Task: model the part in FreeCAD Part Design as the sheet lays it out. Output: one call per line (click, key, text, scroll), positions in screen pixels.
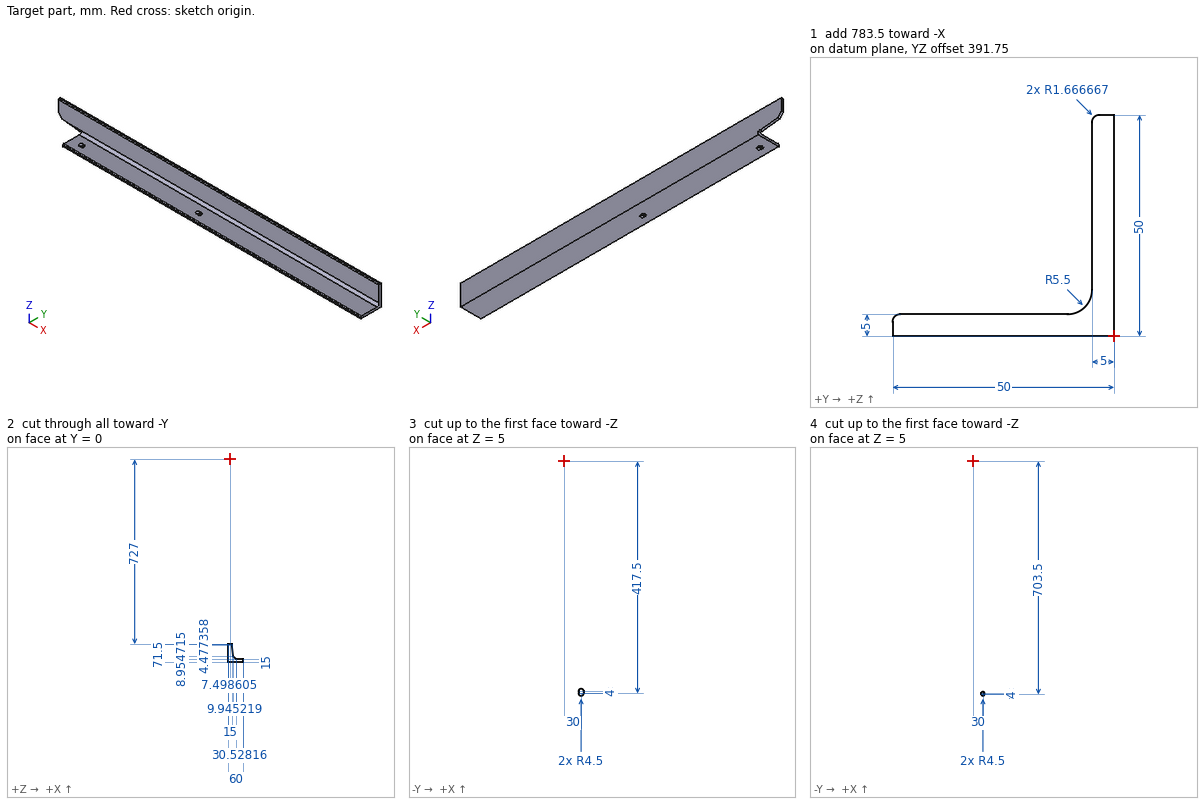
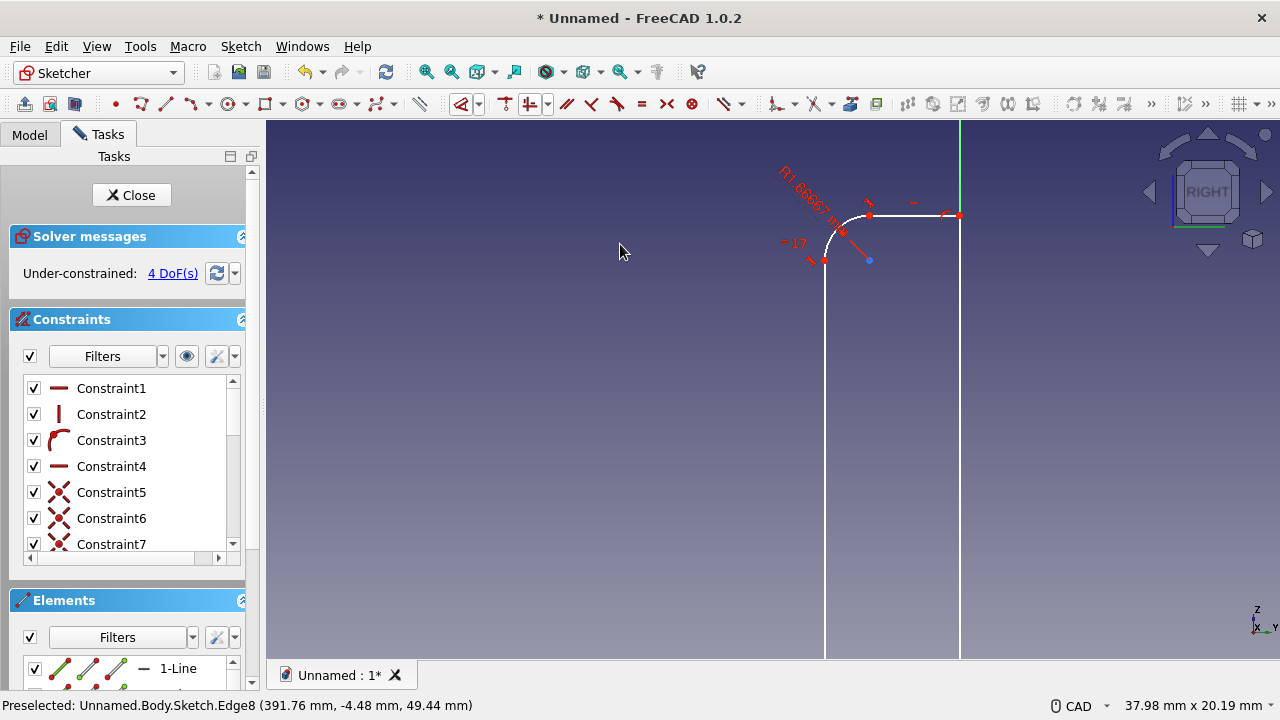
scroll(839, 229, down, 7)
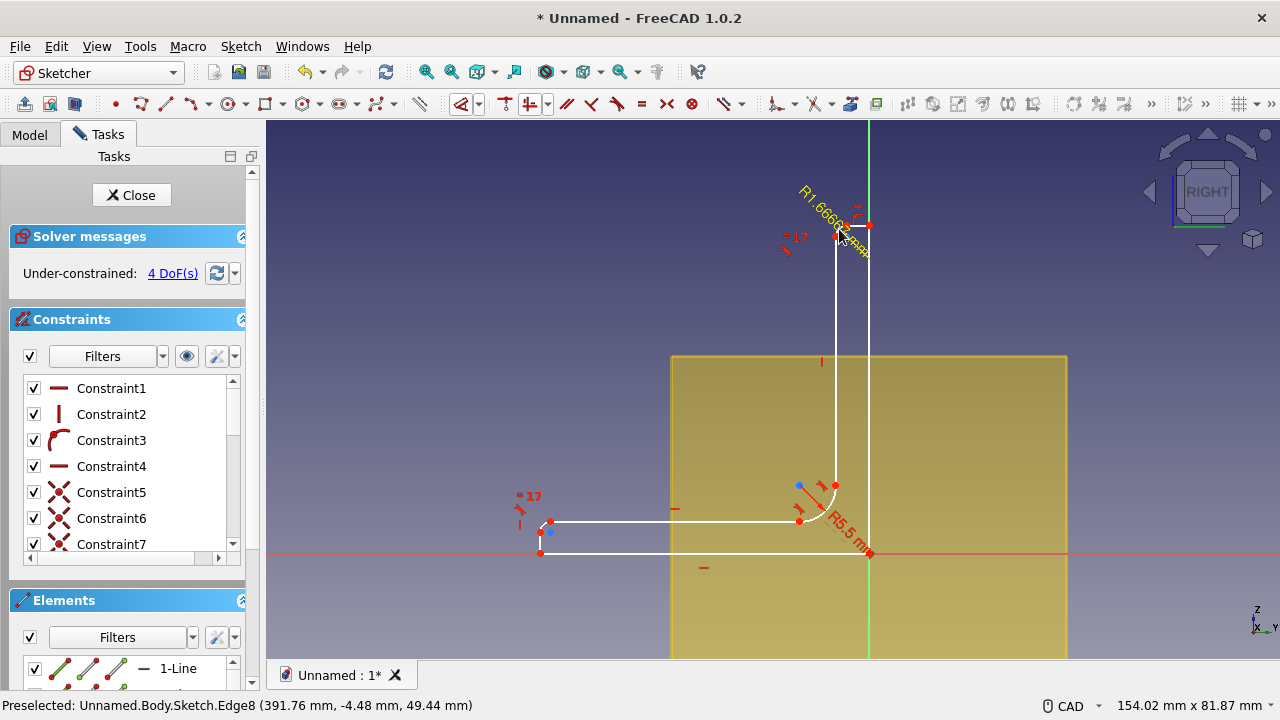
click(869, 324)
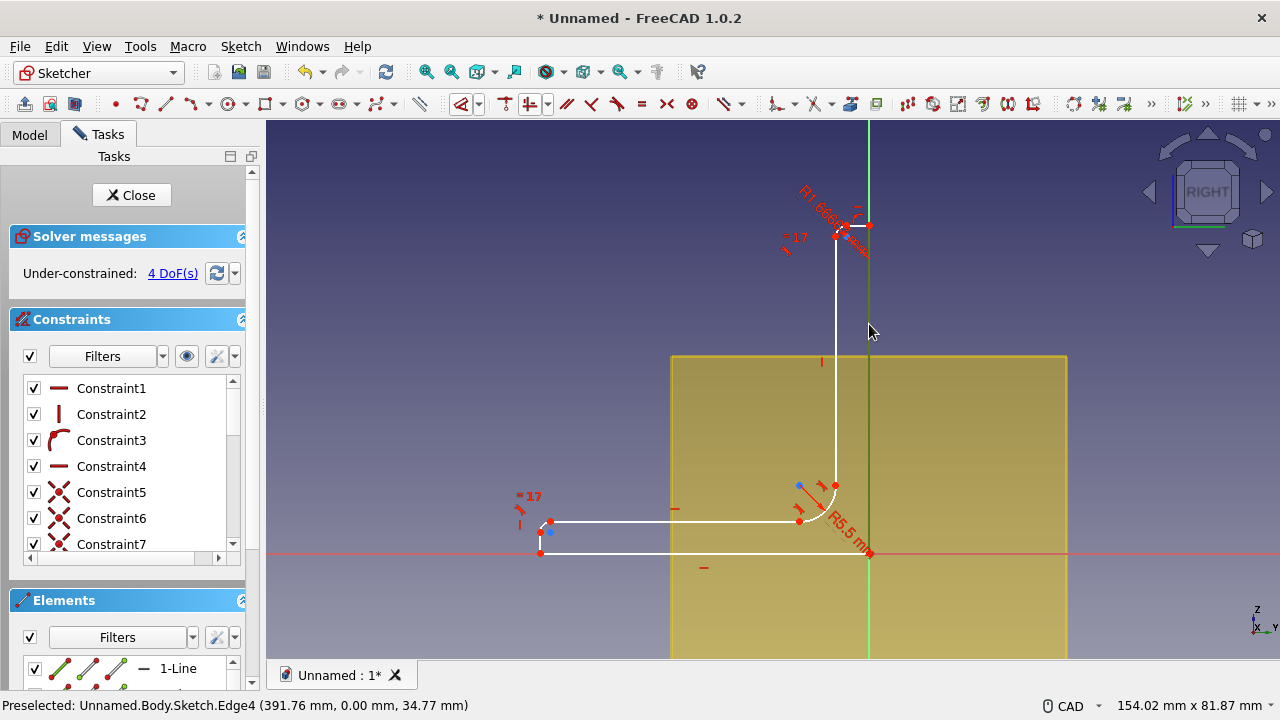
key(i)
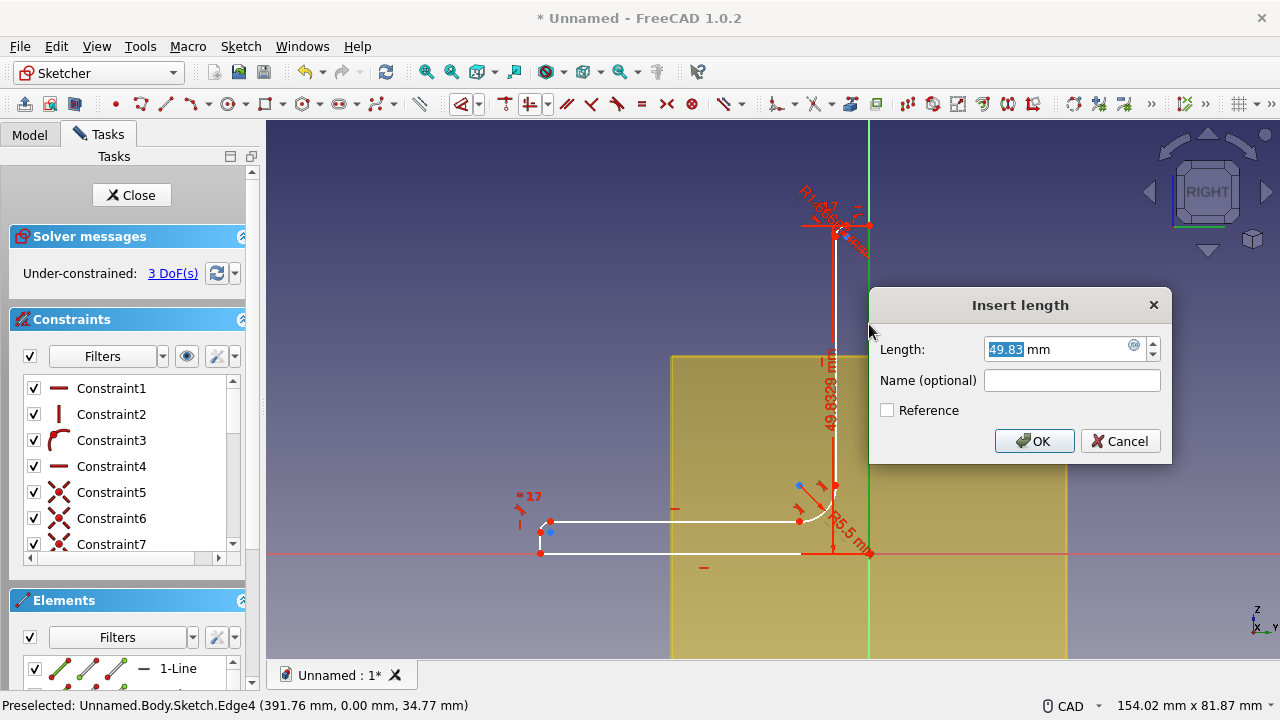
text(50)
key(Return)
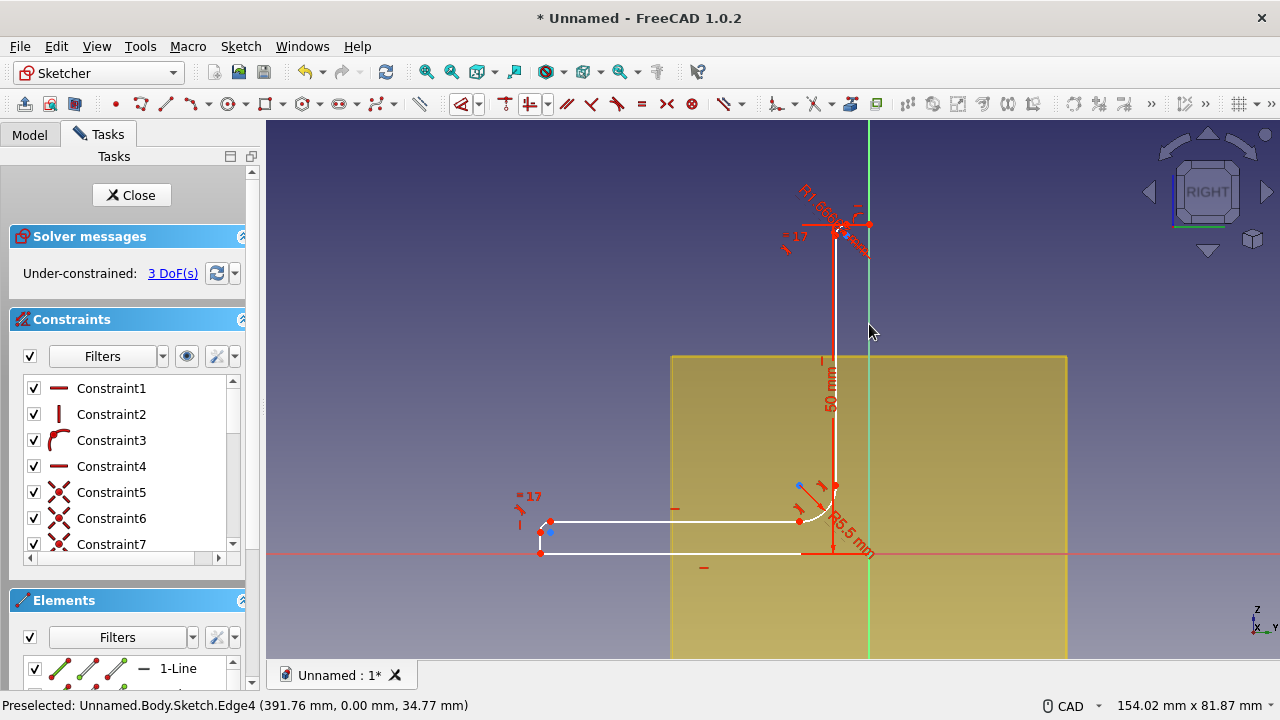
click(770, 554)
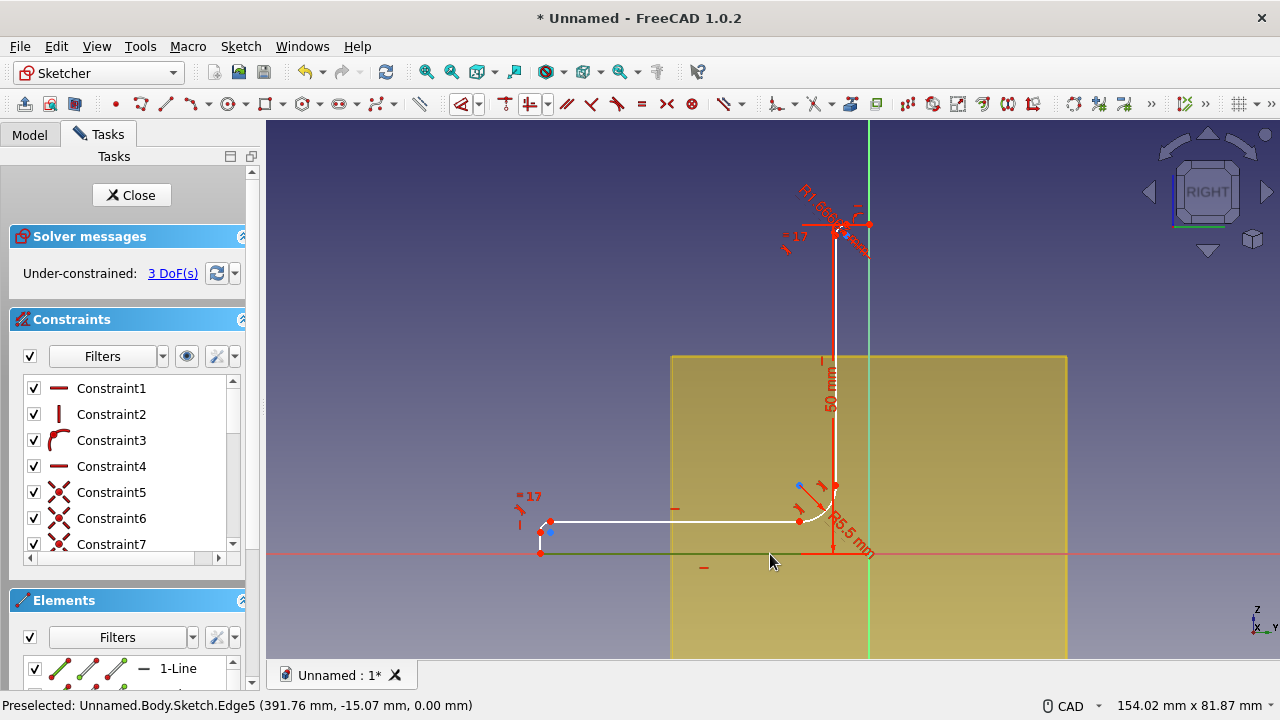
key(l)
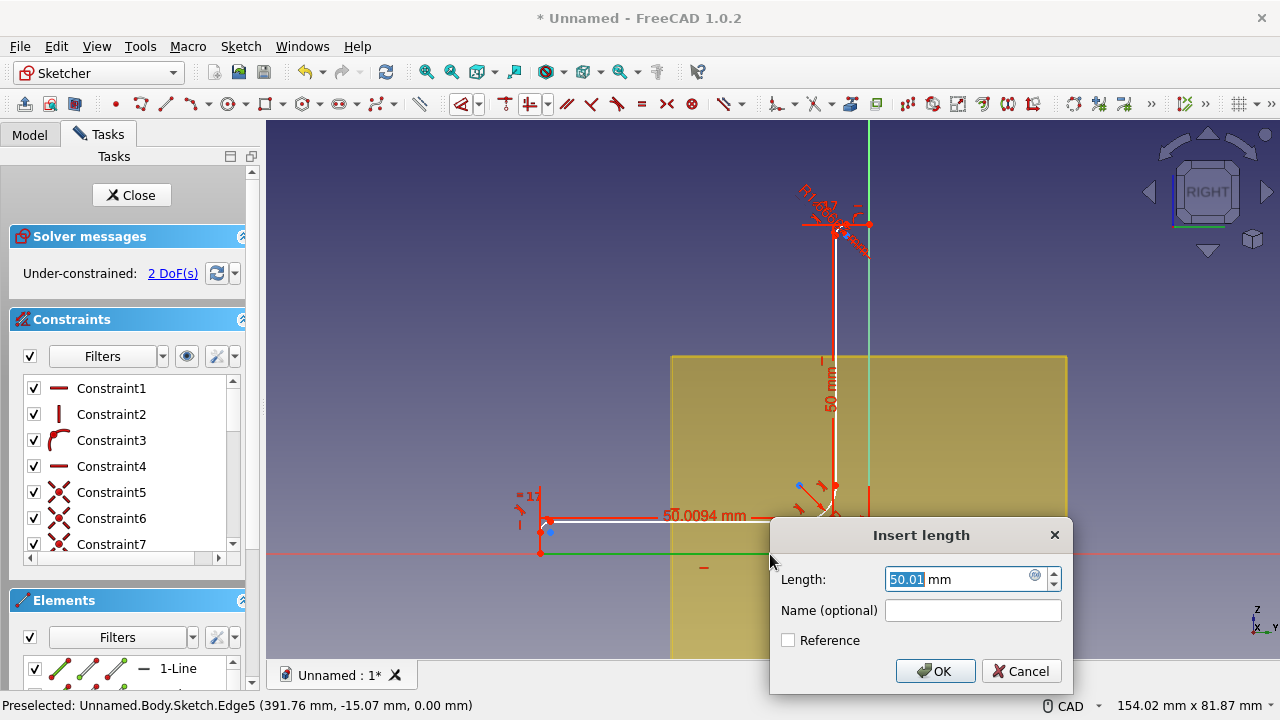
text(50)
key(Return)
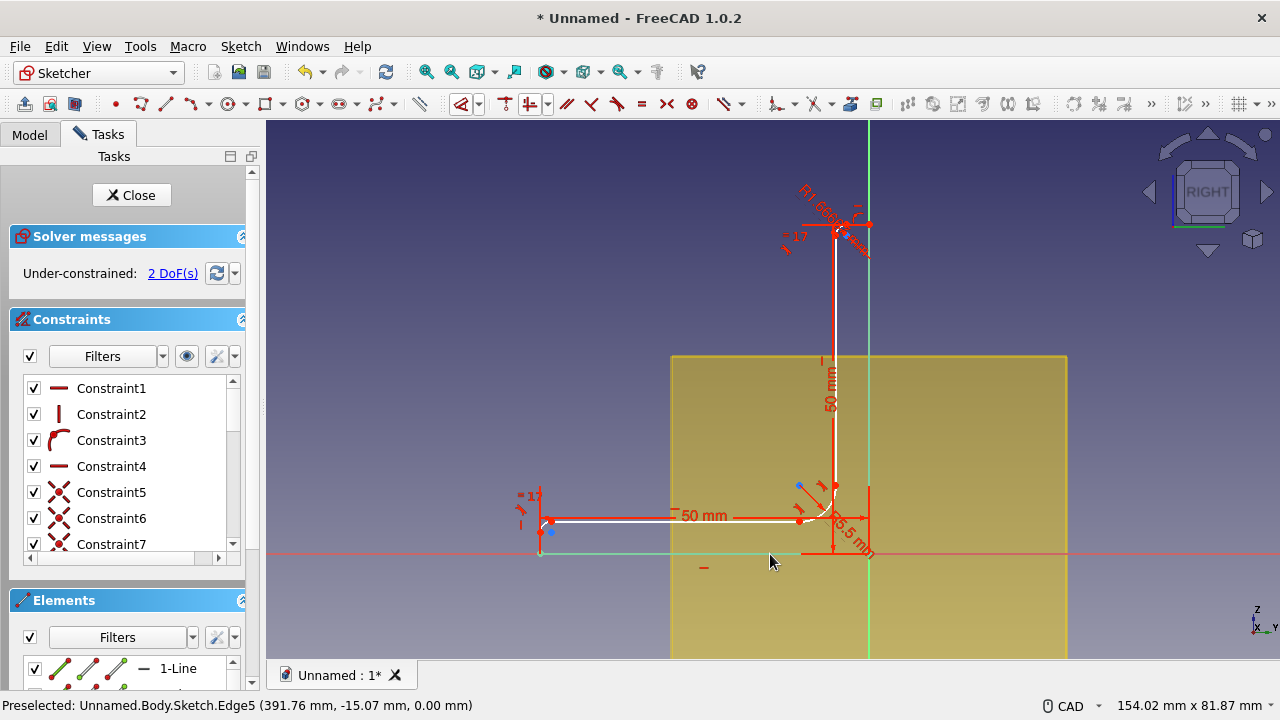
click(551, 522)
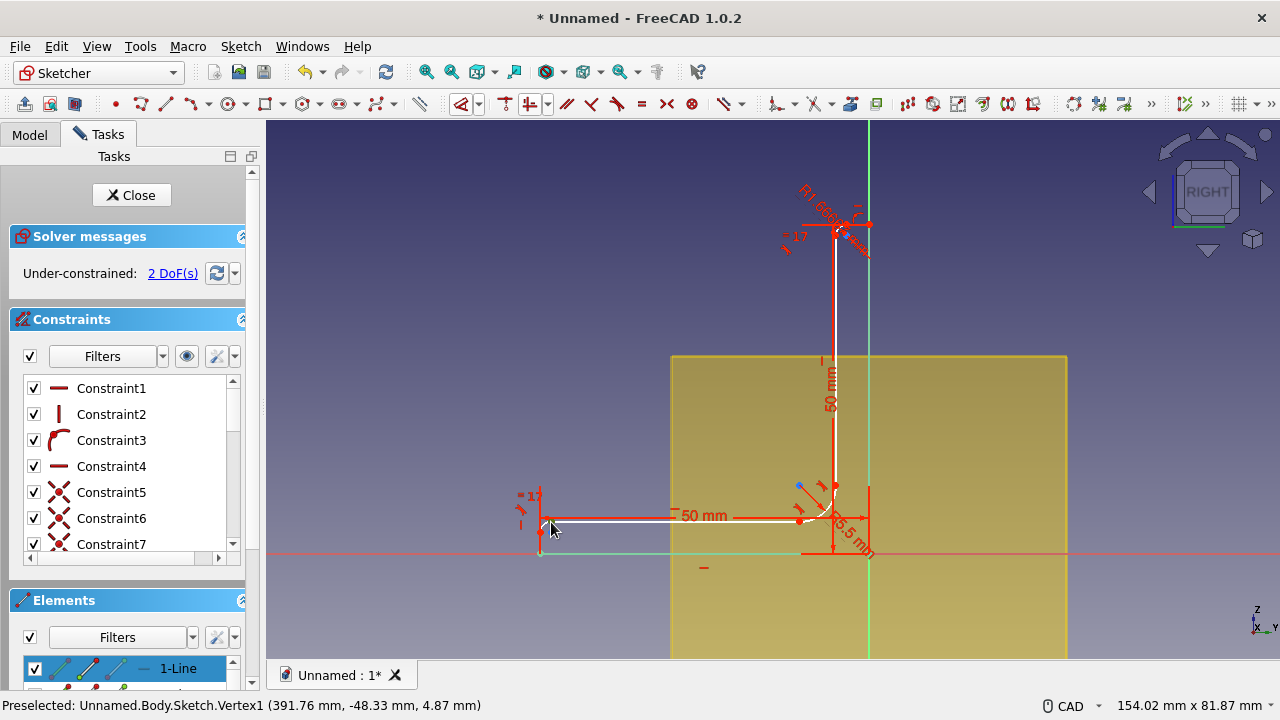
key(i)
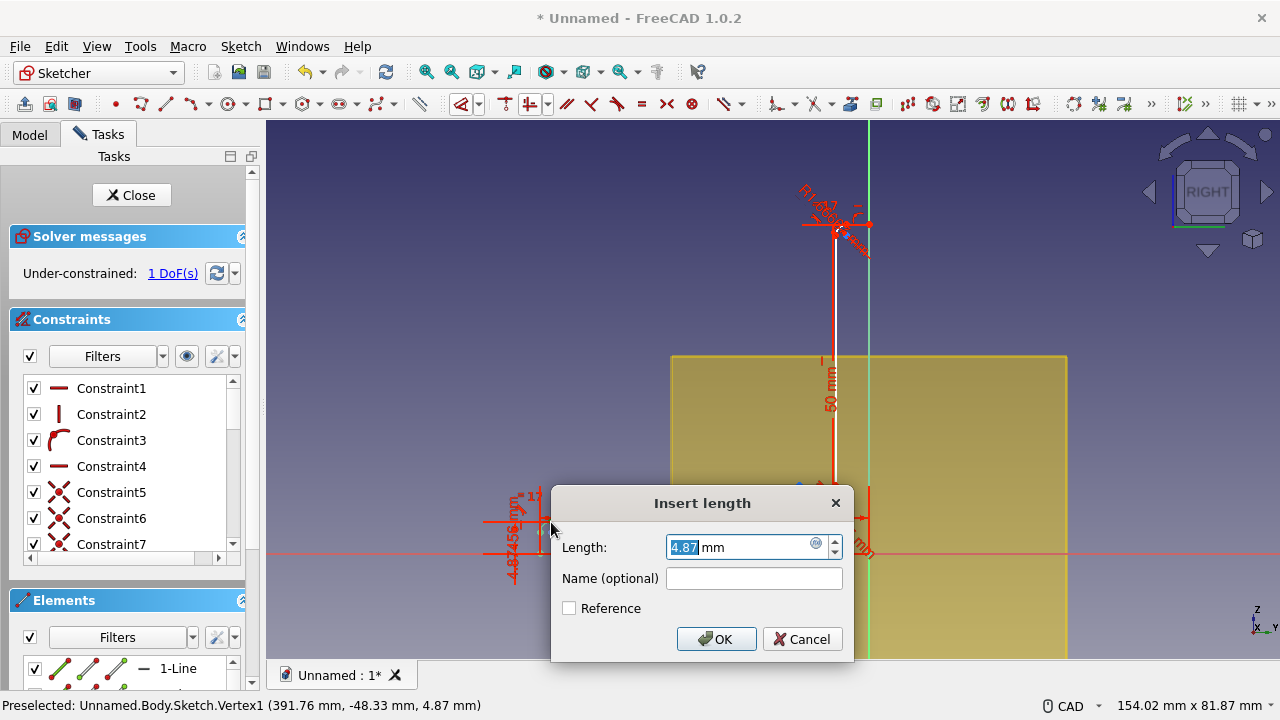
text(5)
key(Return)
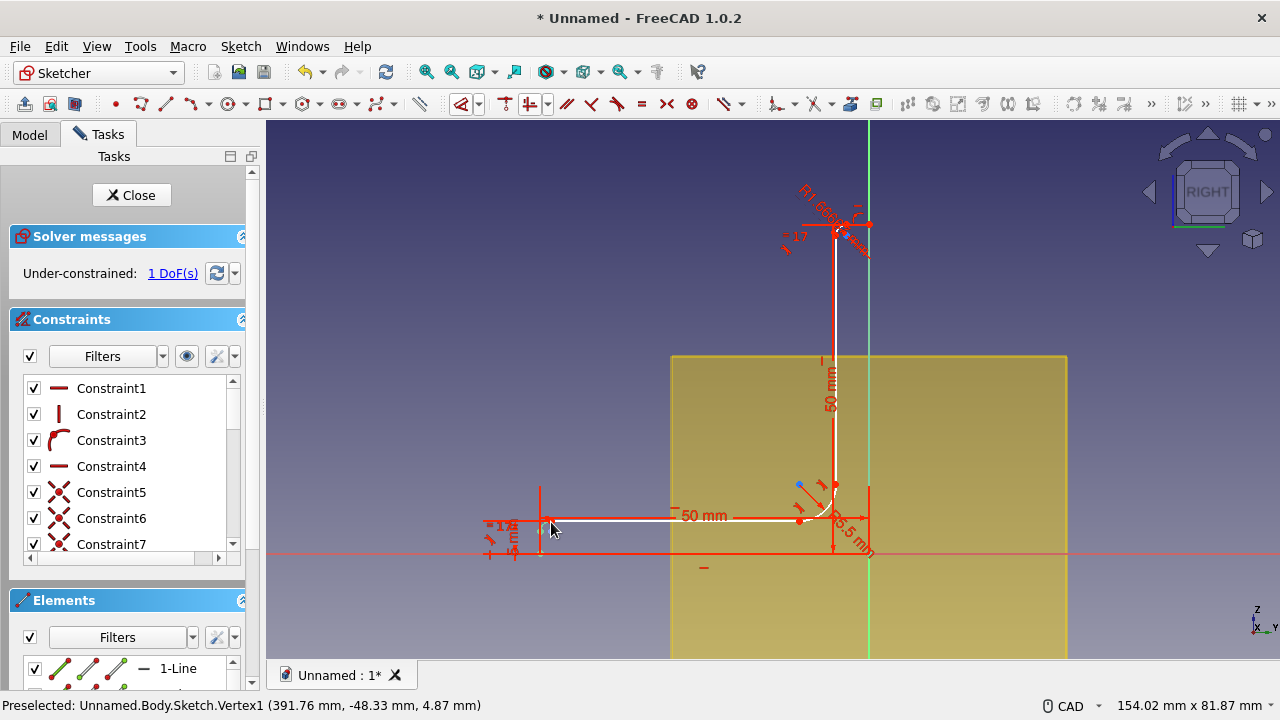
click(836, 485)